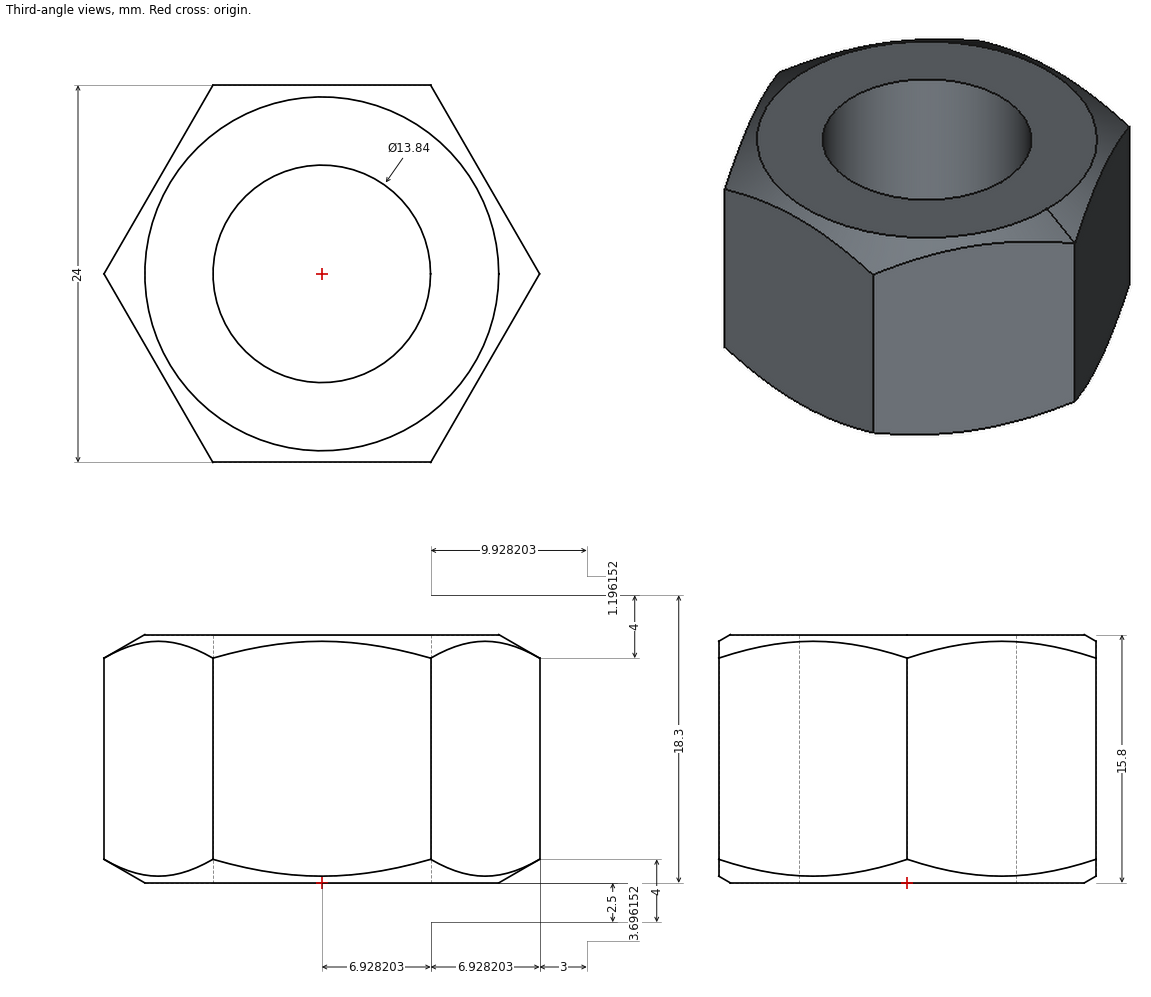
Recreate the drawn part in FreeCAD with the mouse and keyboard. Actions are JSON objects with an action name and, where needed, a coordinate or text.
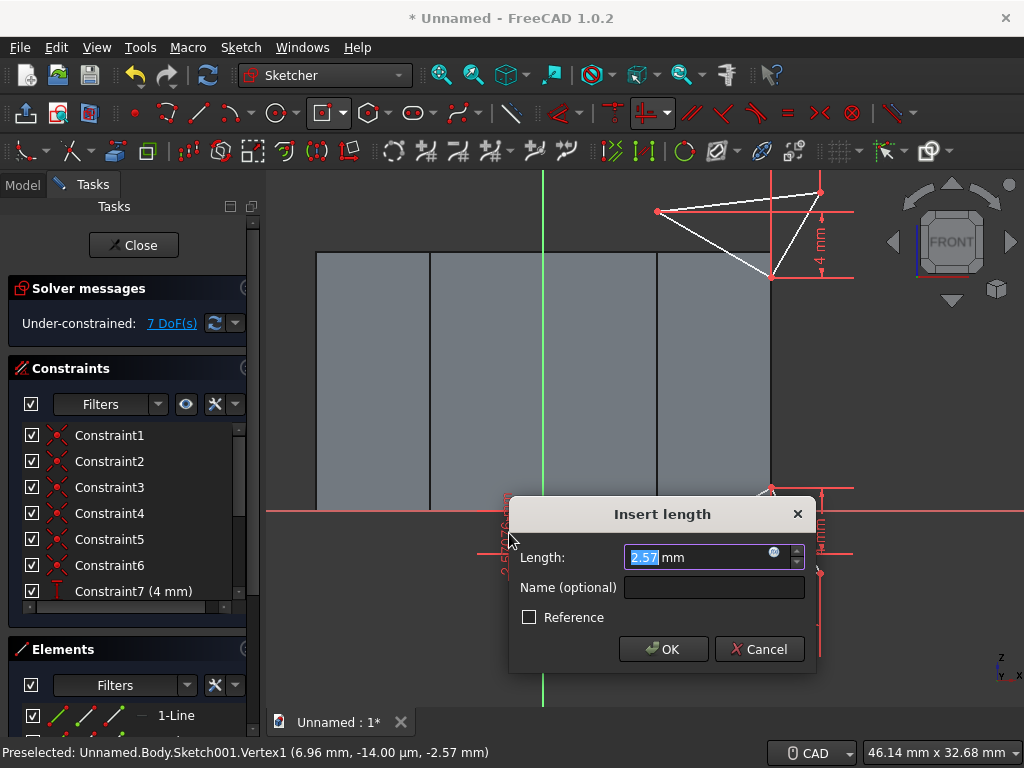
{"action": "type", "text": "2.5"}
{"action": "key", "text": "Return"}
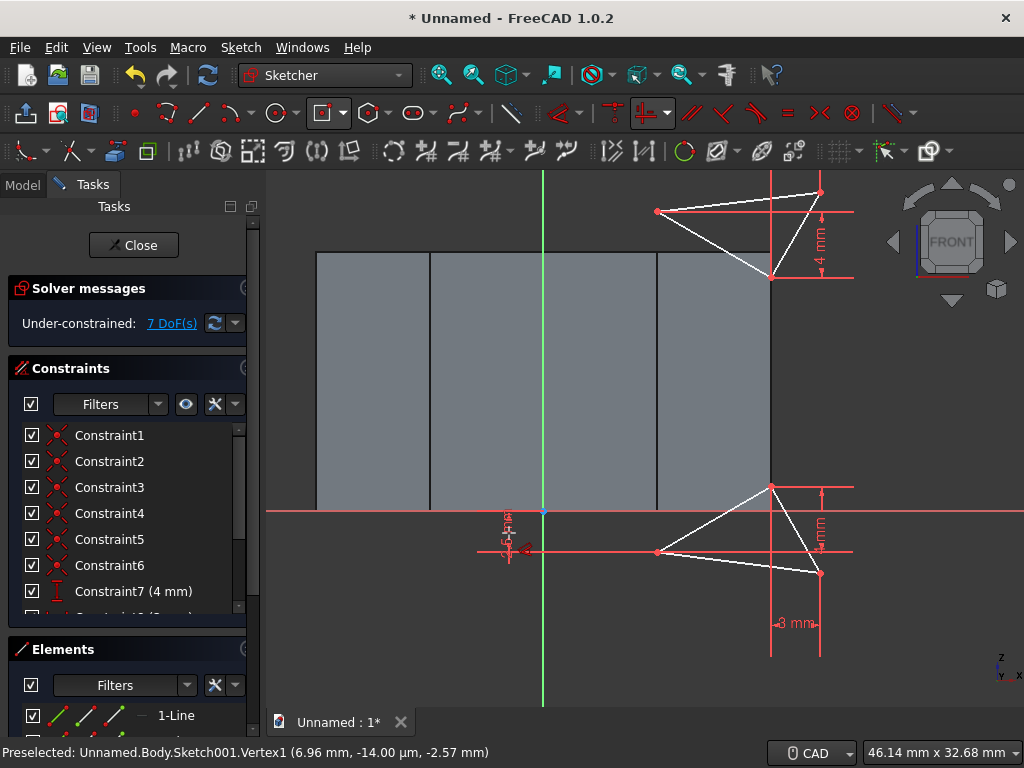
{"action": "left_click", "coordinate": [658, 212]}
{"action": "left_click", "coordinate": [509, 362]}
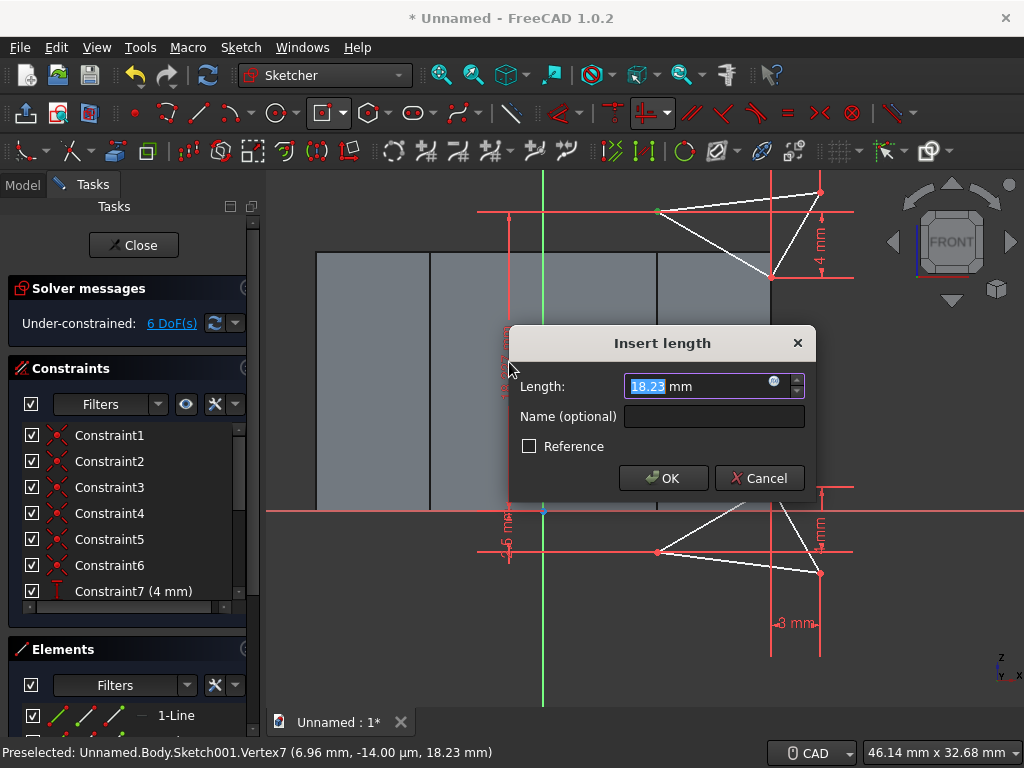
{"action": "type", "text": "18.3"}
{"action": "key", "text": "Return"}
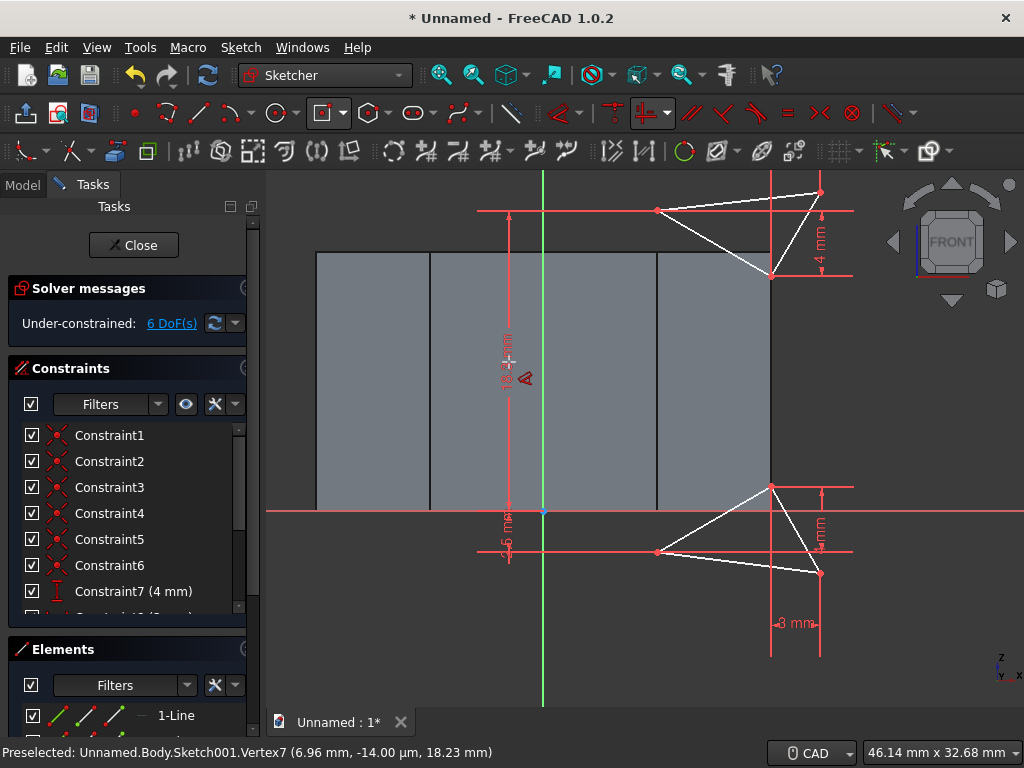
{"action": "left_click", "coordinate": [658, 552]}
{"action": "left_click", "coordinate": [601, 586]}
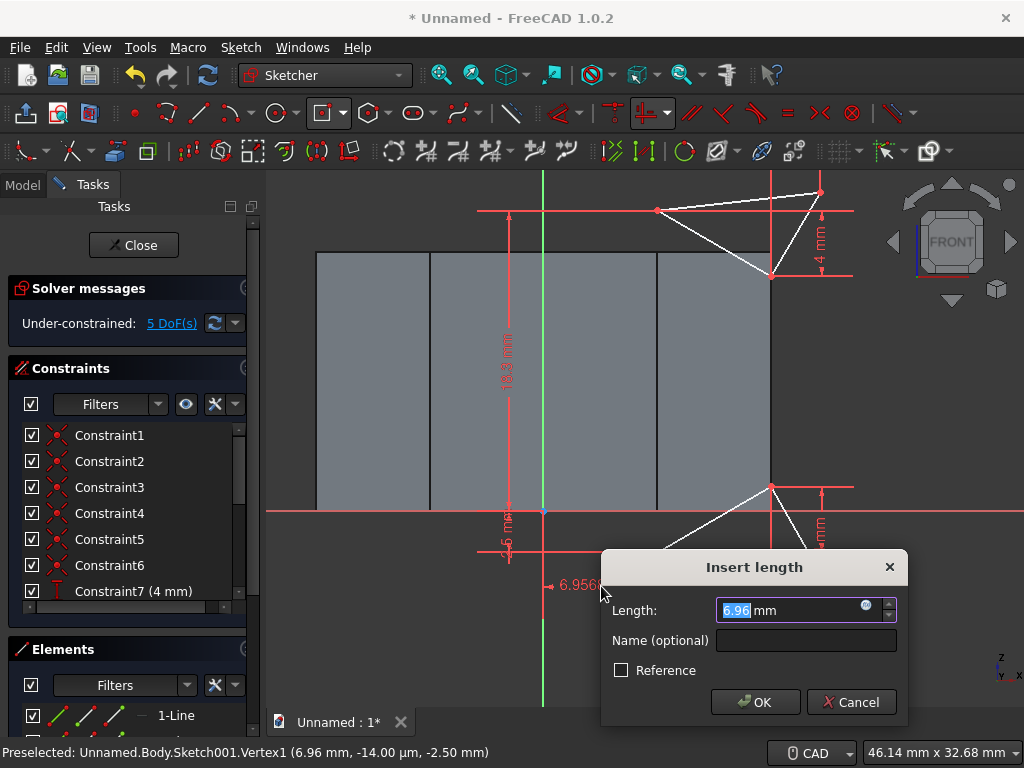
{"action": "type", "text": "6.928203"}
{"action": "key", "text": "Return"}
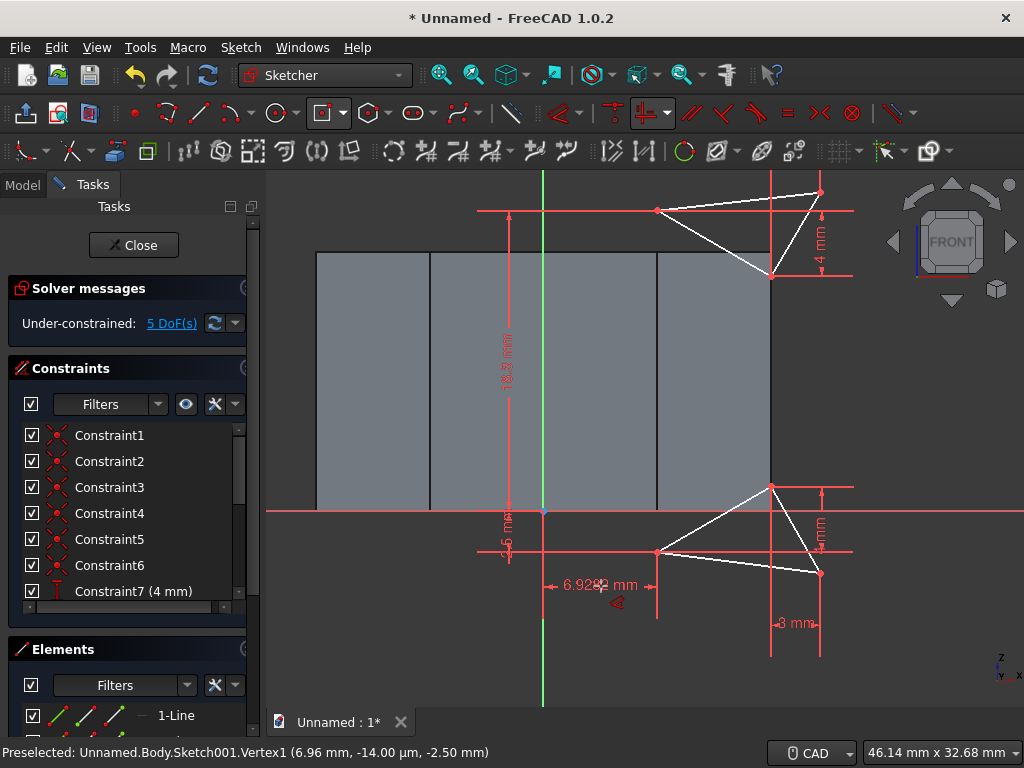
{"action": "left_click", "coordinate": [820, 573]}
{"action": "left_click", "coordinate": [509, 556]}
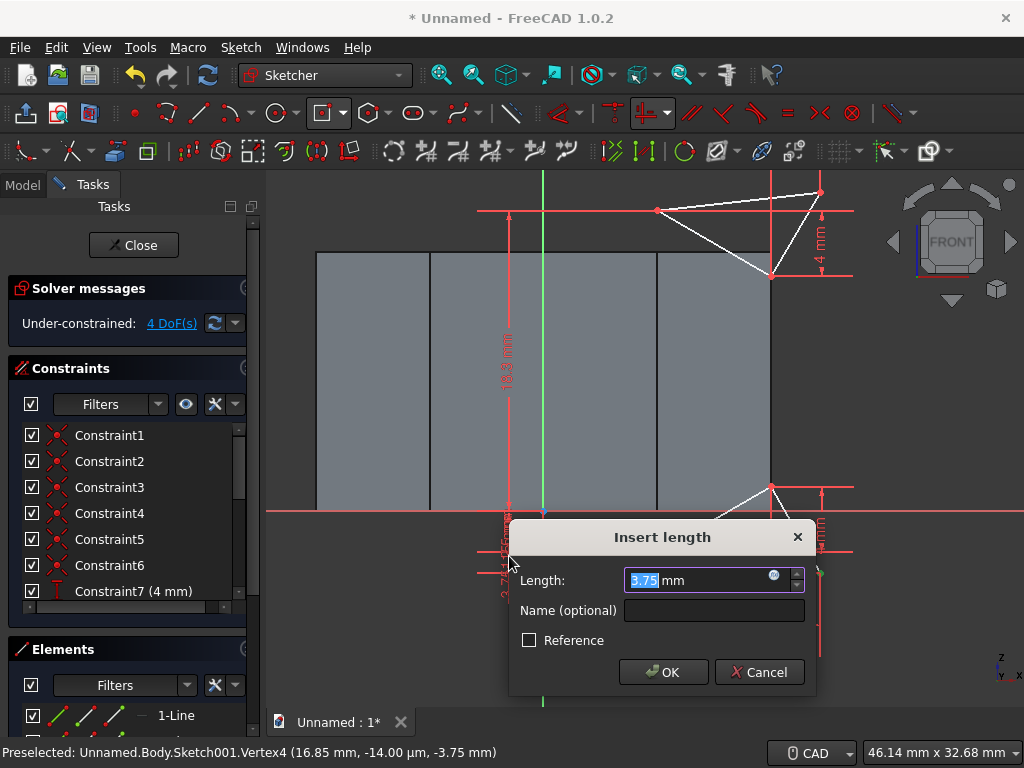
{"action": "type", "text": "3.696152"}
{"action": "key", "text": "Return"}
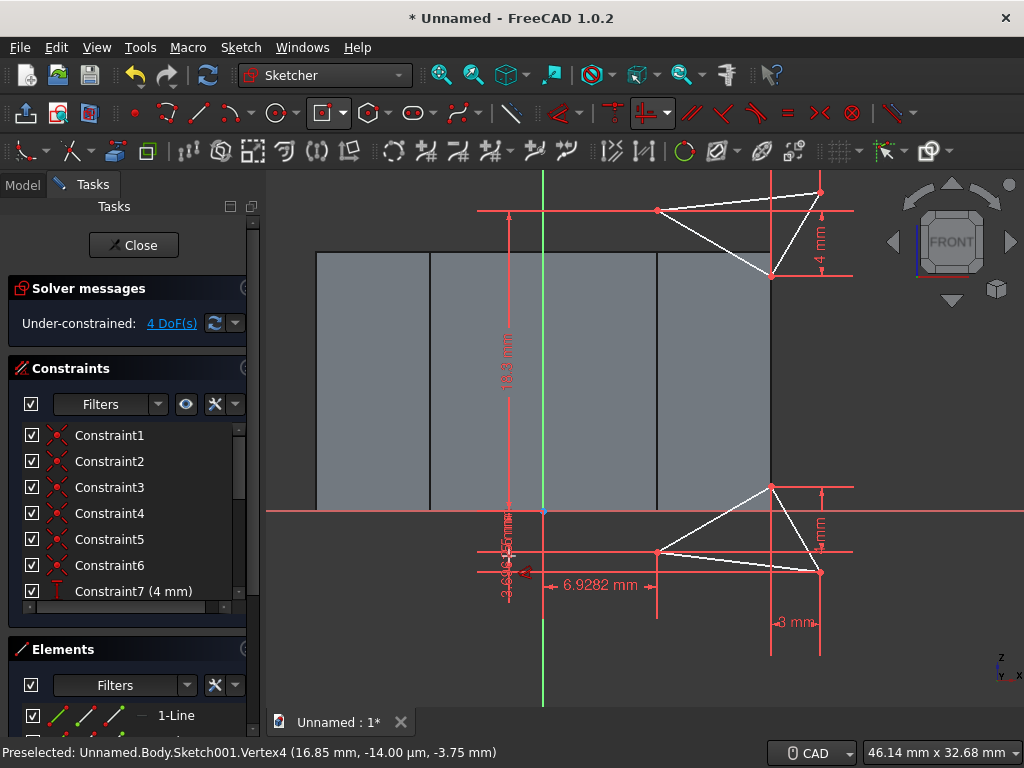
{"action": "left_click", "coordinate": [658, 211]}
{"action": "left_click", "coordinate": [601, 545]}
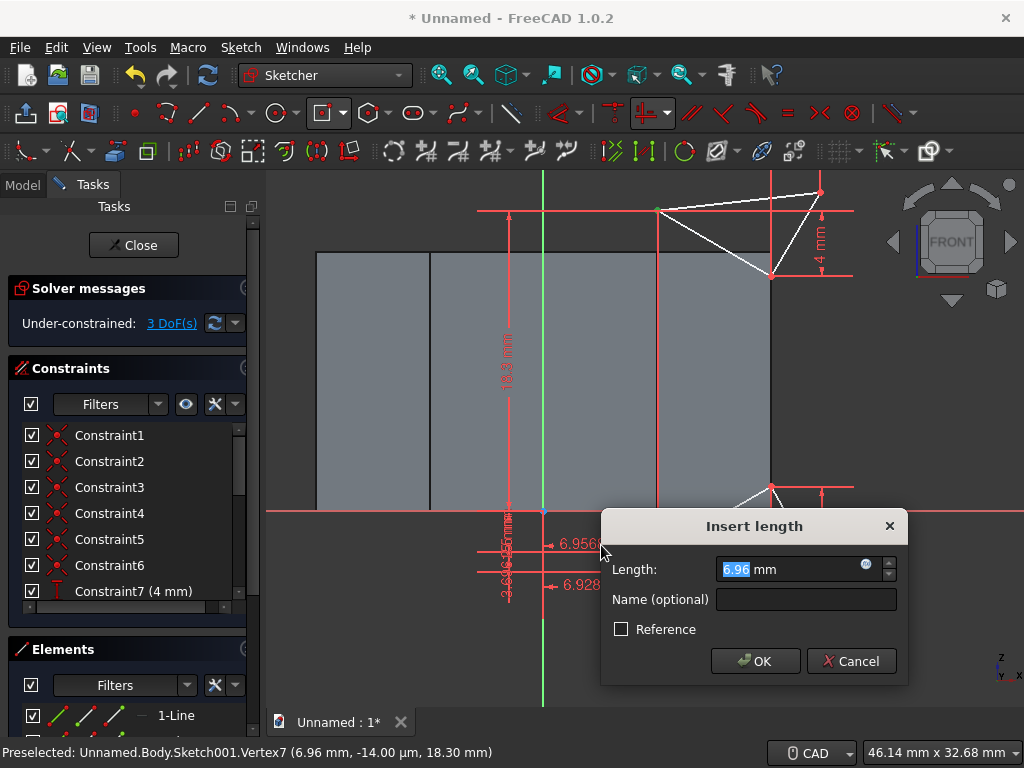
{"action": "type", "text": "6.928203"}
{"action": "key", "text": "Return"}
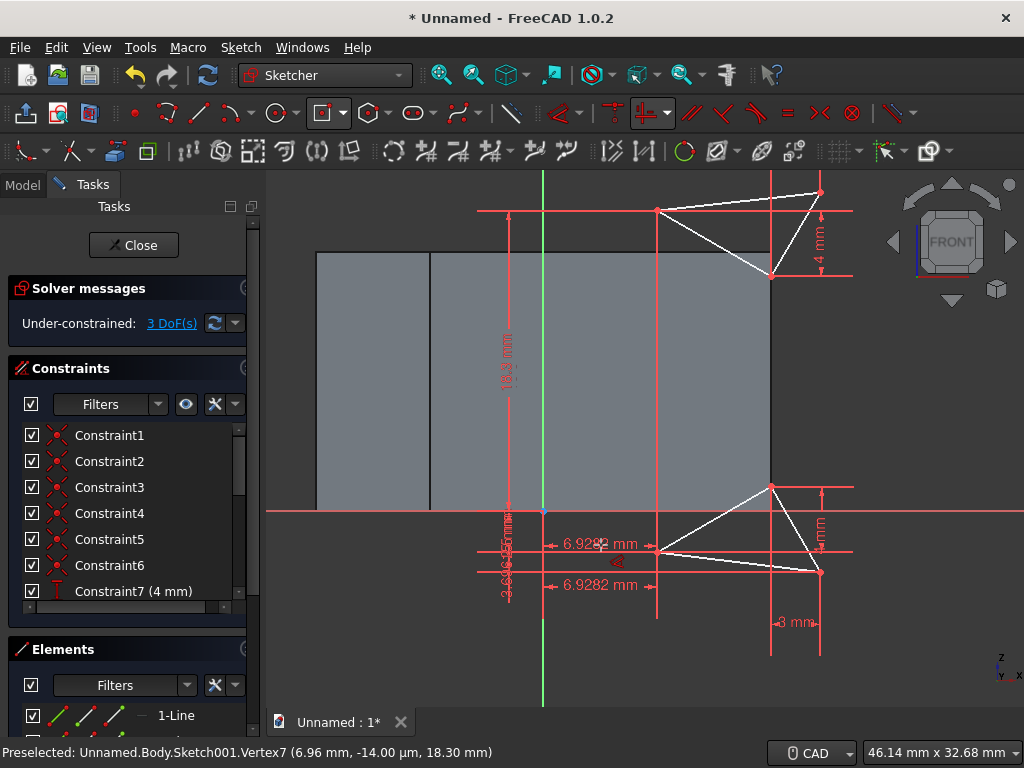
{"action": "left_click", "coordinate": [691, 533]}
{"action": "left_click", "coordinate": [714, 586]}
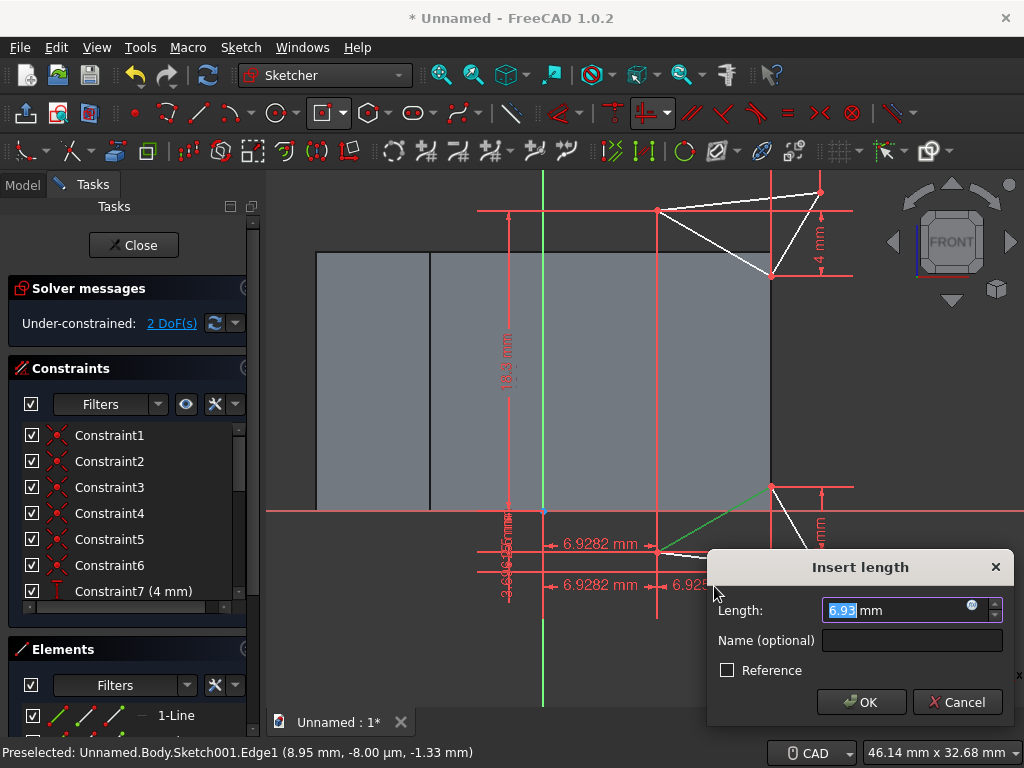
{"action": "type", "text": "6.928203"}
{"action": "key", "text": "Return"}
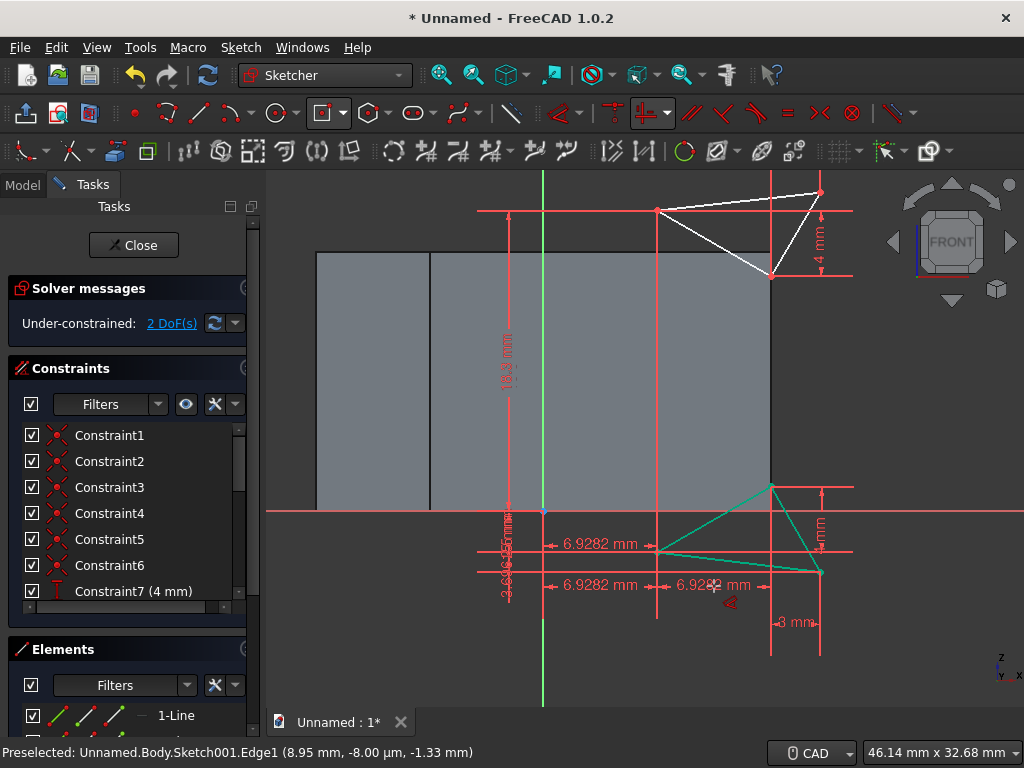
{"action": "left_click", "coordinate": [706, 205]}
{"action": "left_click", "coordinate": [682, 245]}